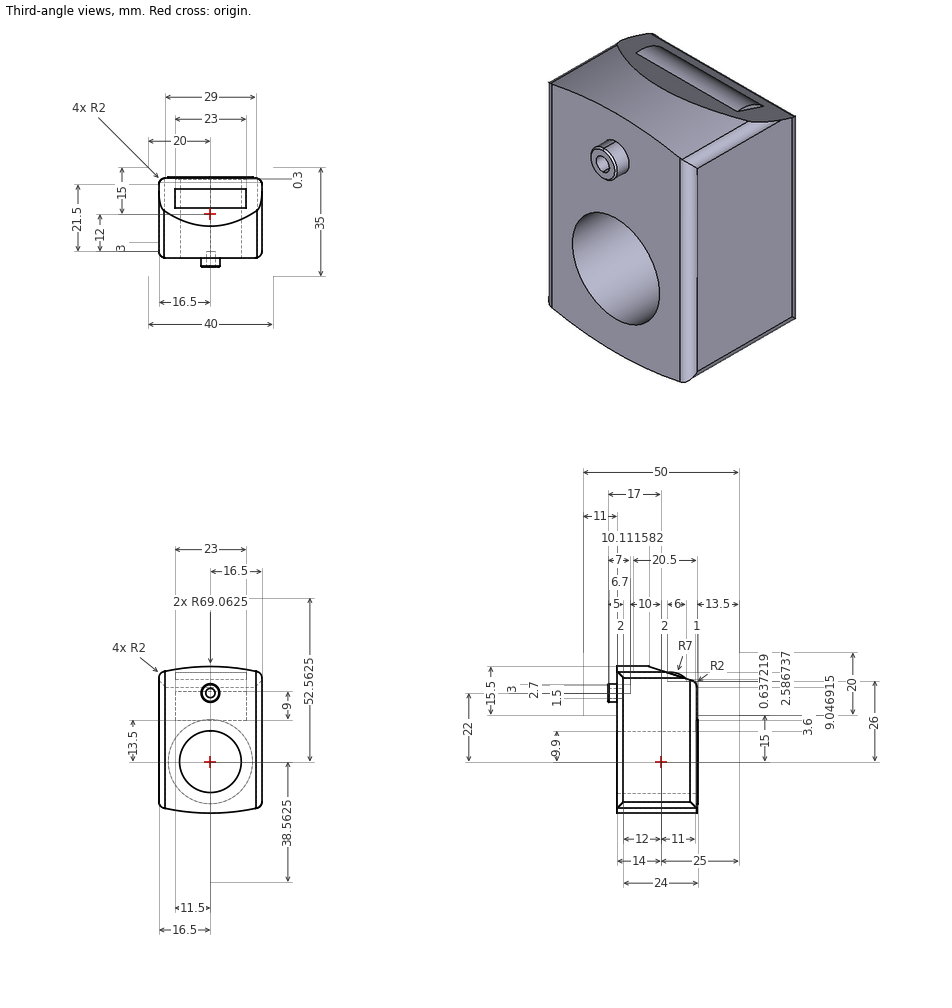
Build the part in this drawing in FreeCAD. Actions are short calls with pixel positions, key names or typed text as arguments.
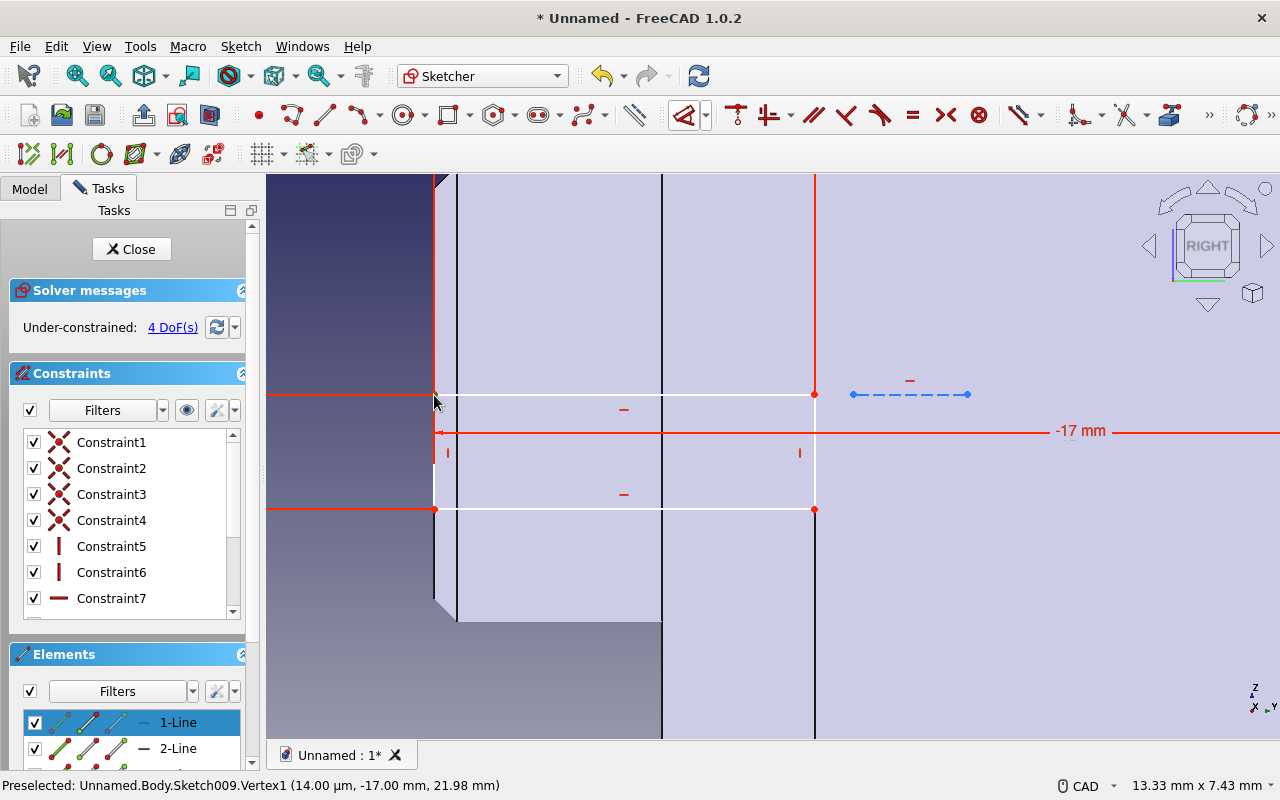
click(706, 116)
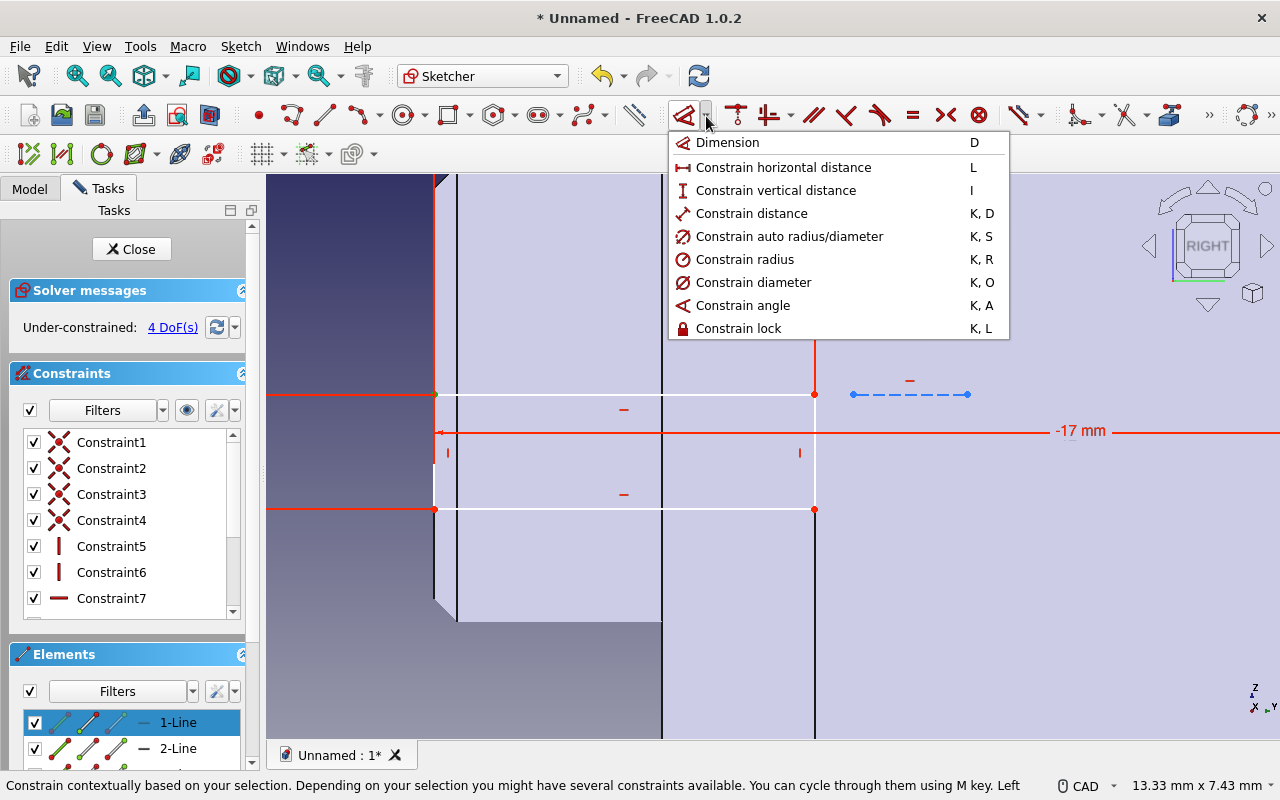
click(839, 190)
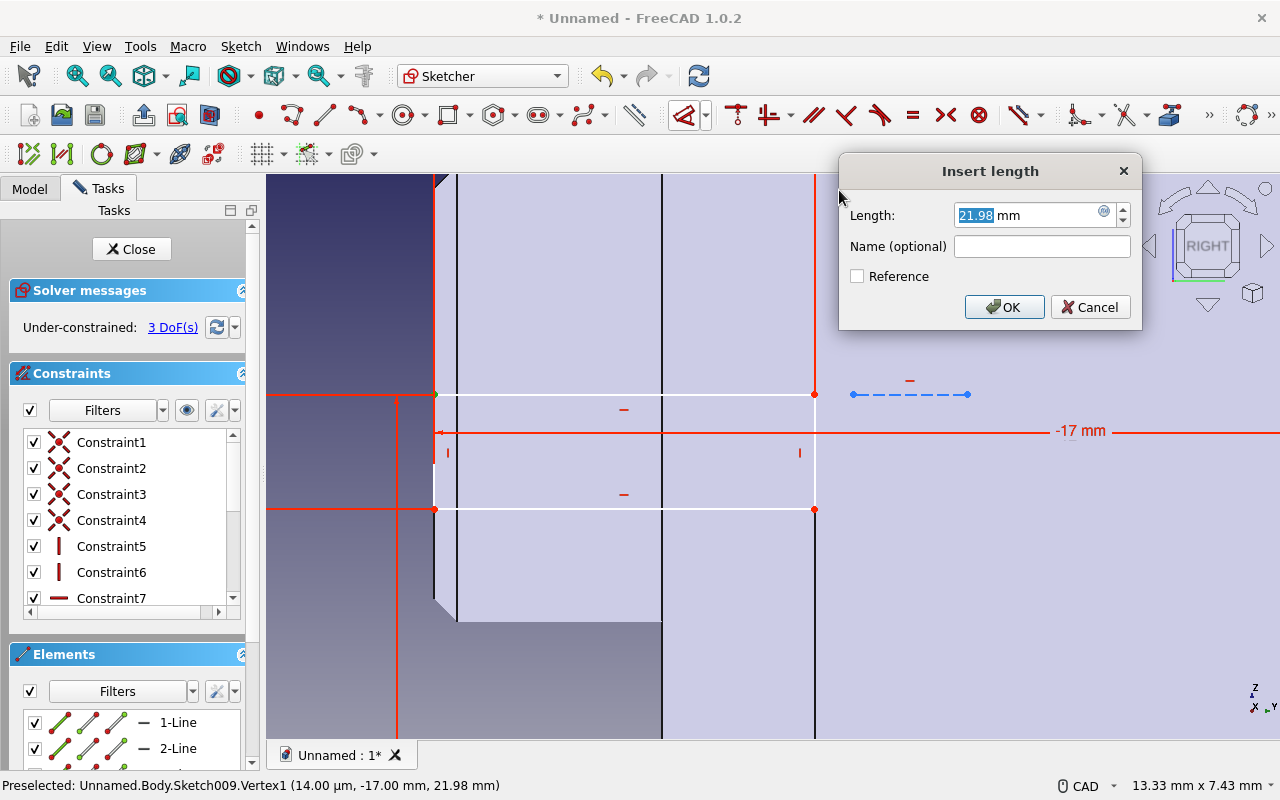
text(22)
key(Return)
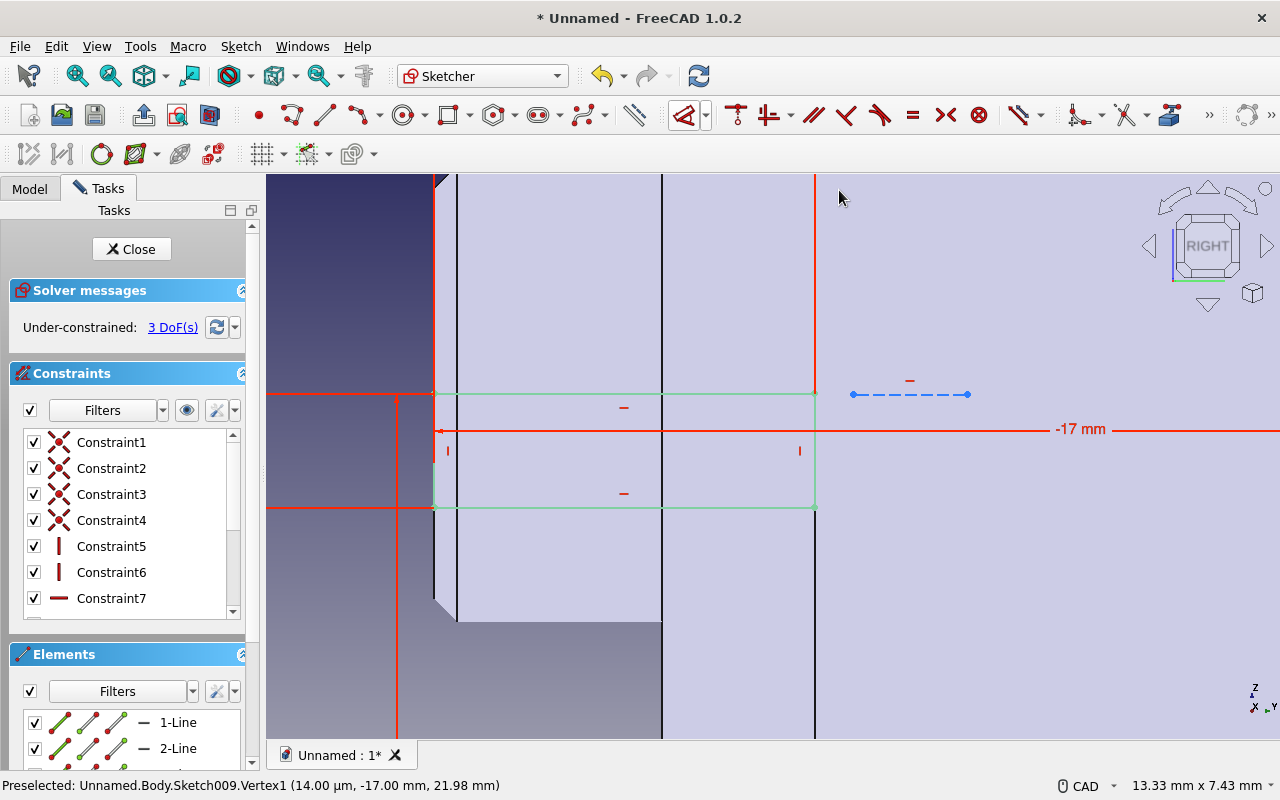
click(853, 395)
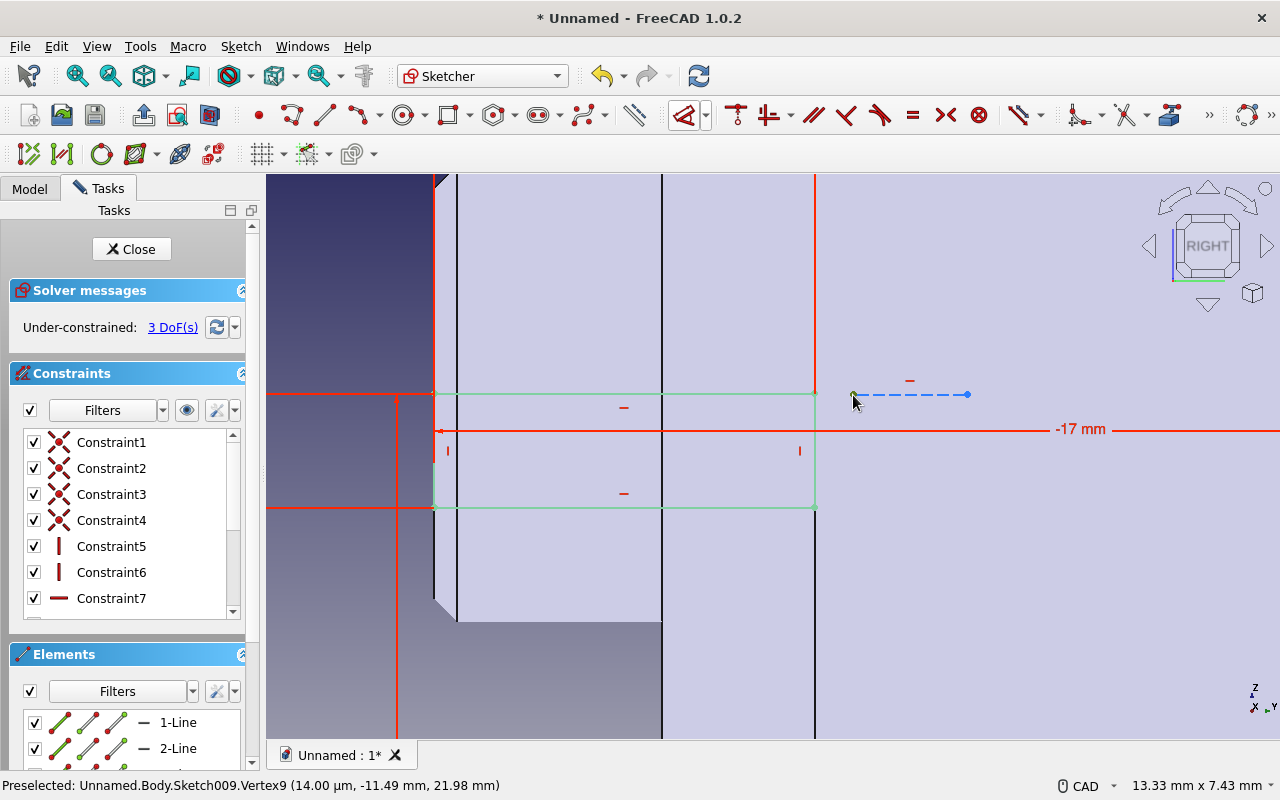
click(706, 116)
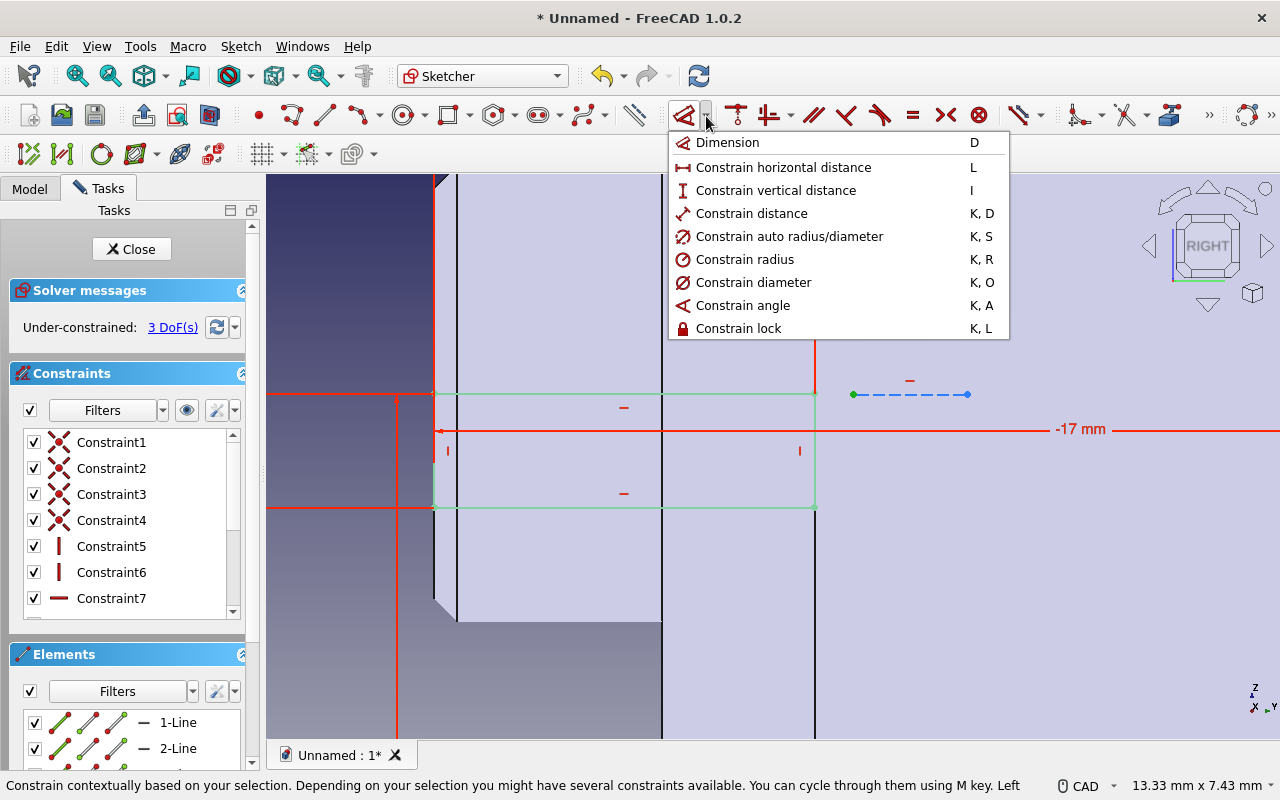
click(839, 190)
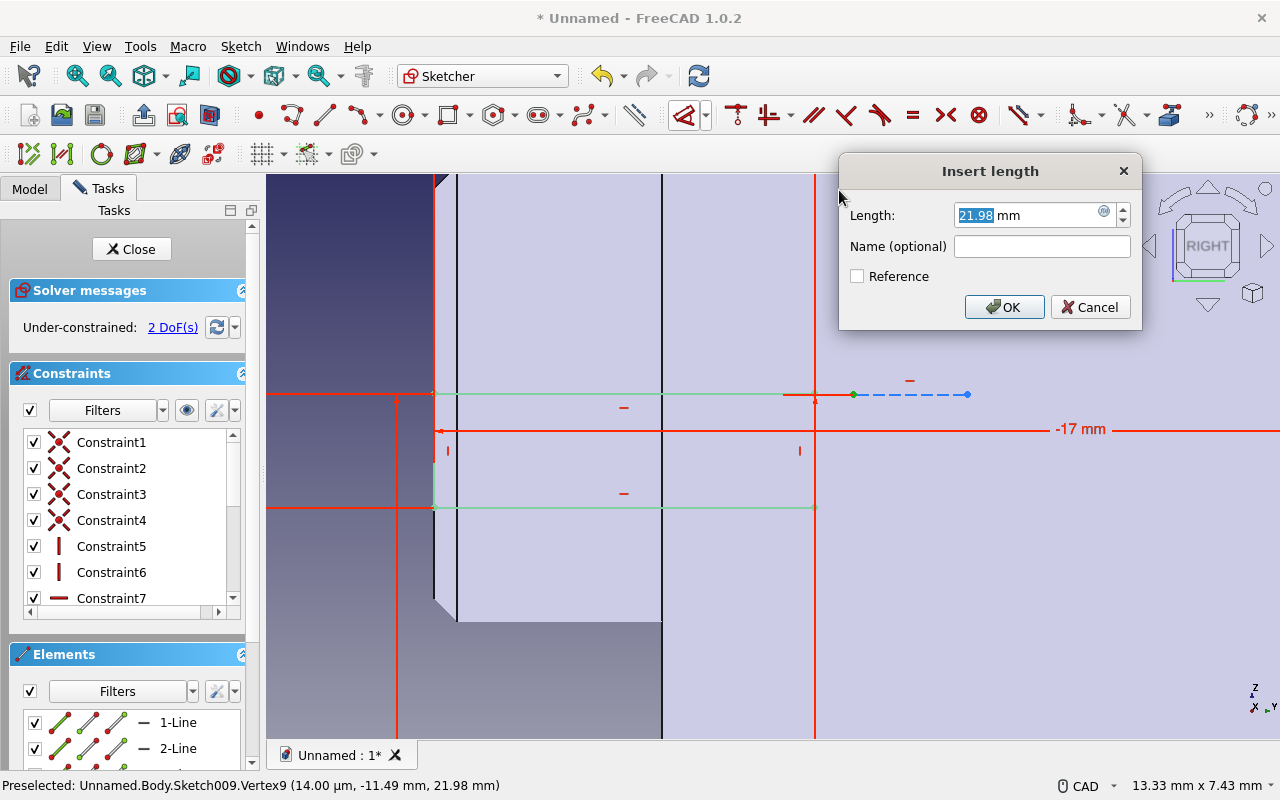
text(22)
key(Return)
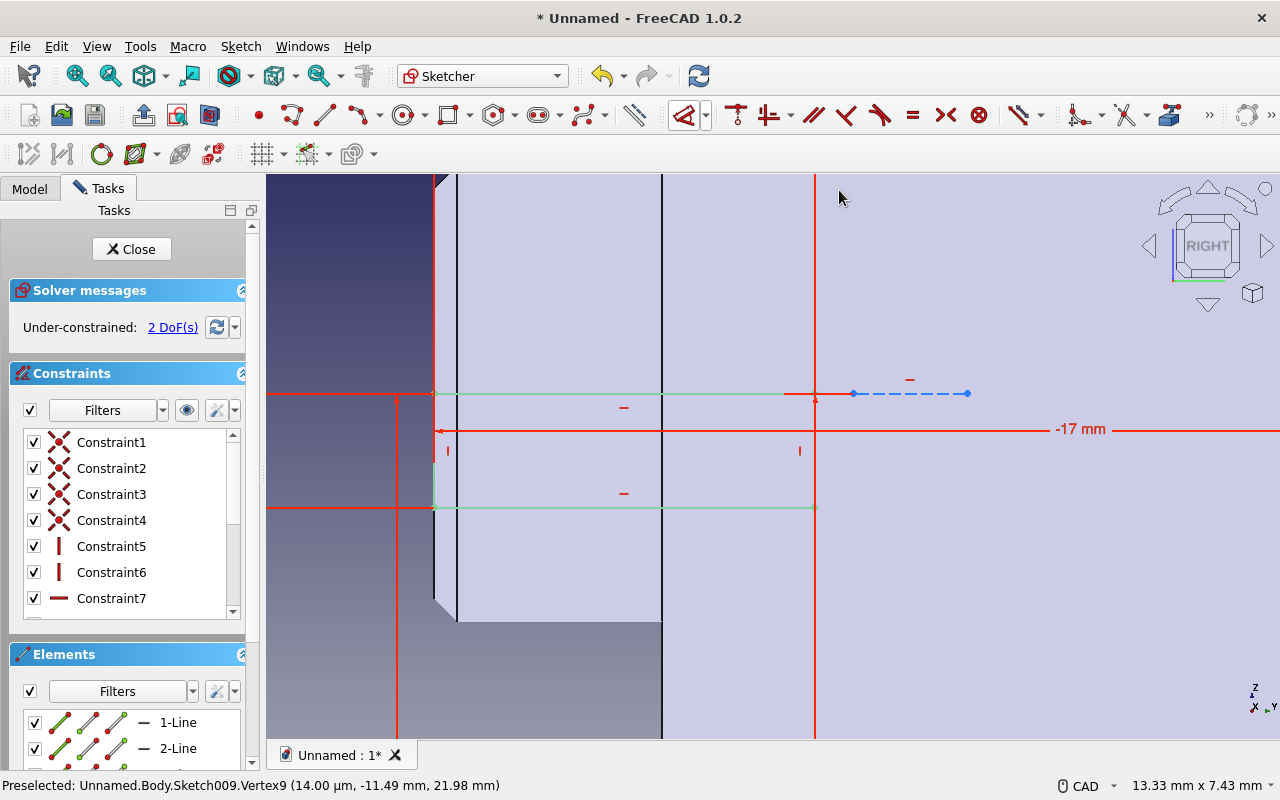
click(132, 249)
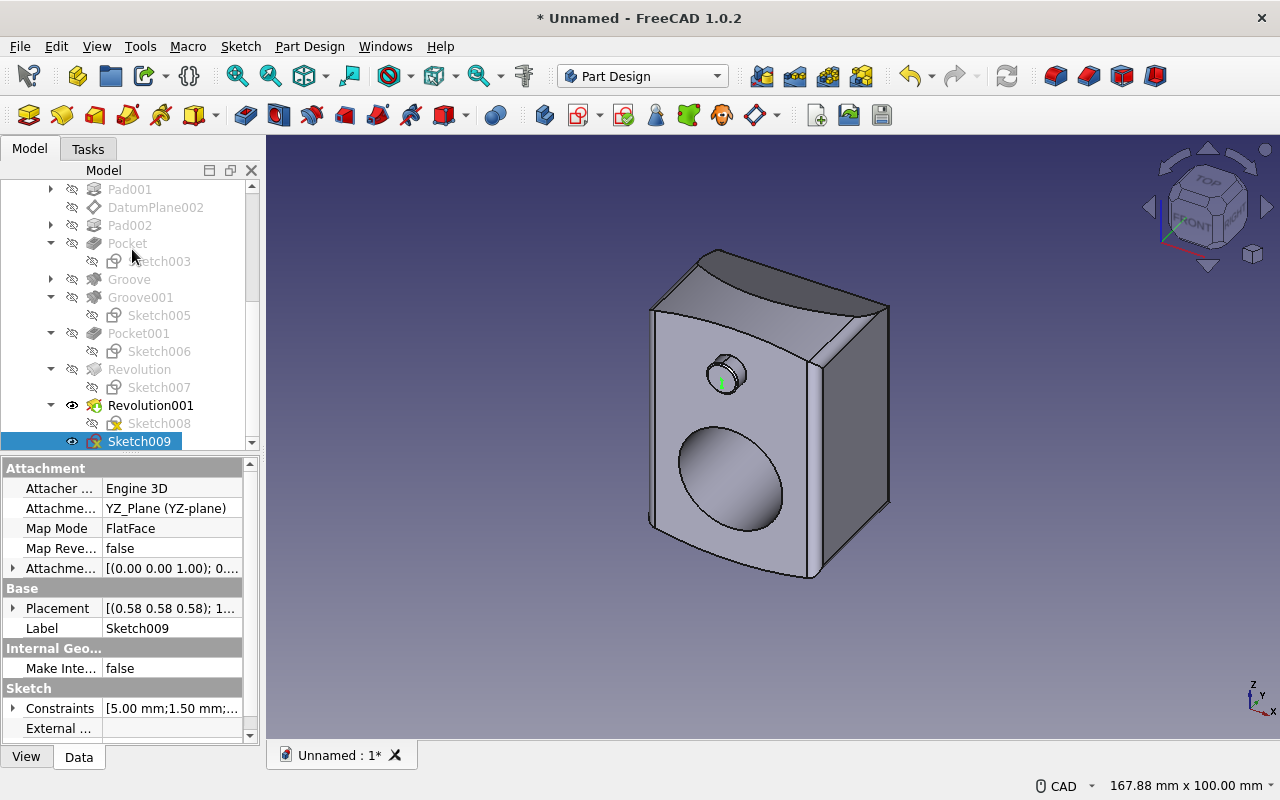
click(312, 116)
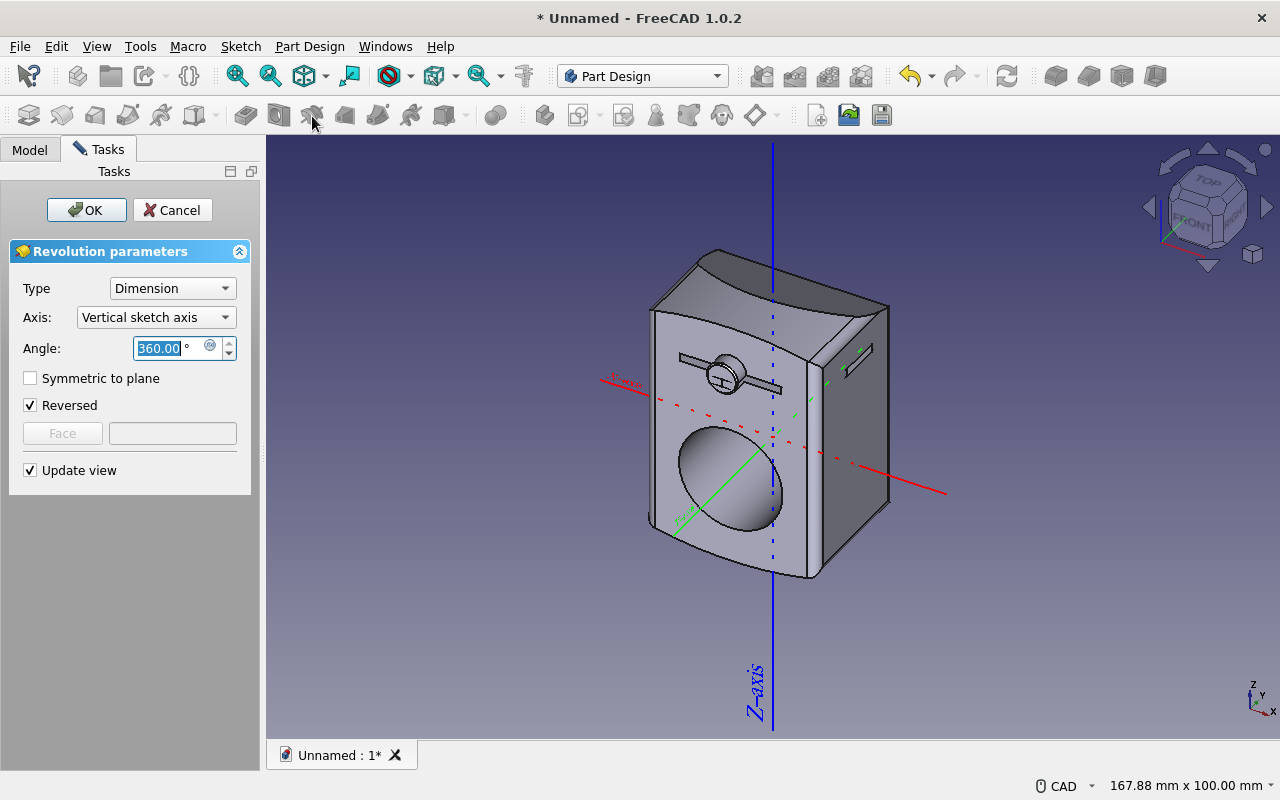
click(157, 318)